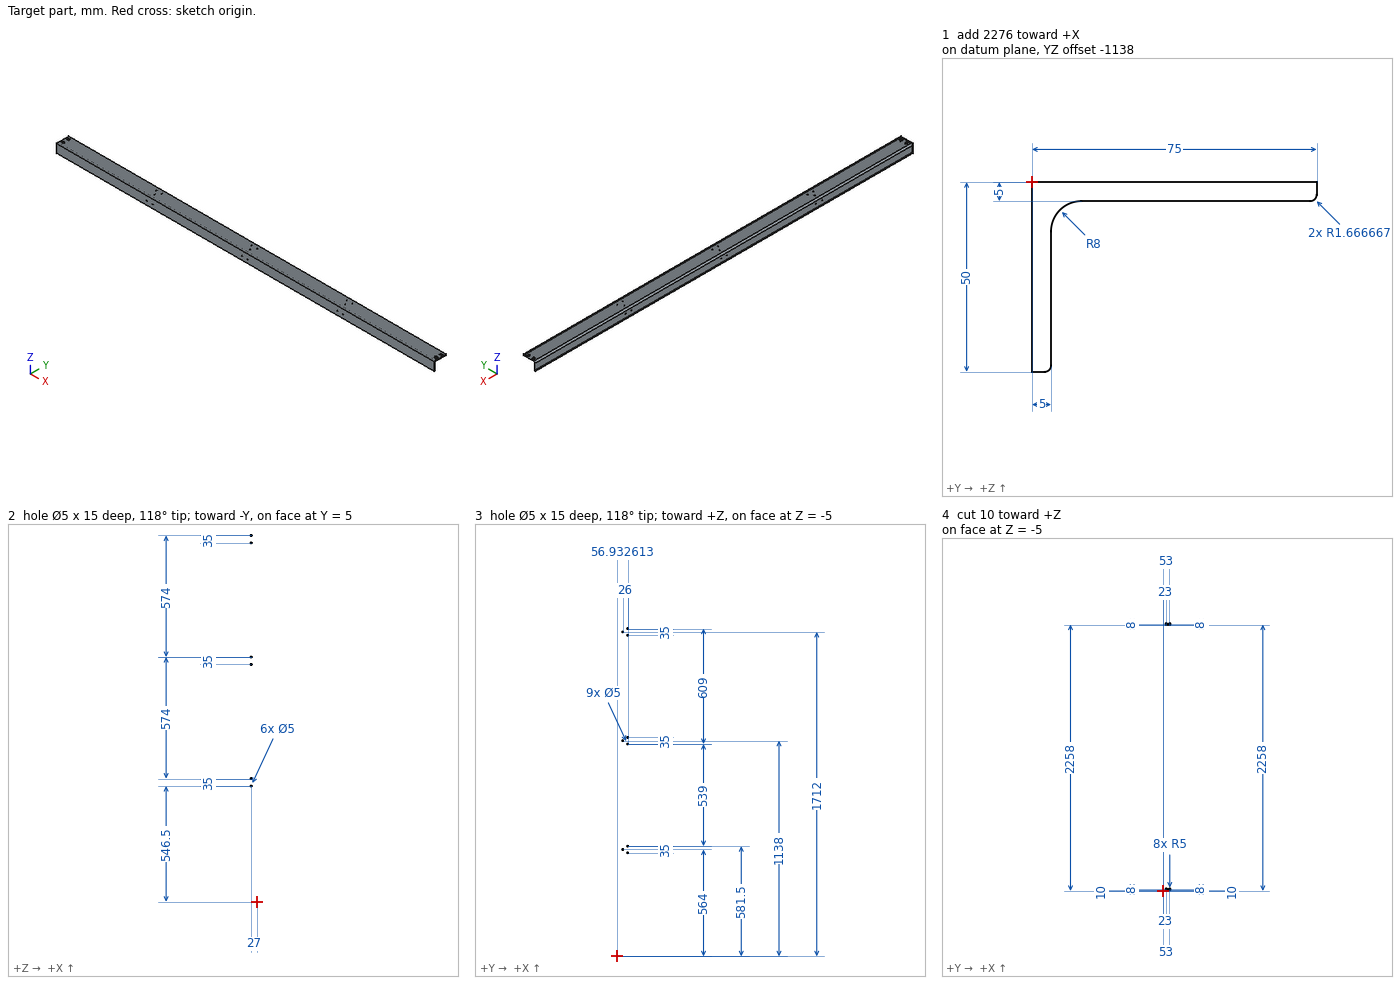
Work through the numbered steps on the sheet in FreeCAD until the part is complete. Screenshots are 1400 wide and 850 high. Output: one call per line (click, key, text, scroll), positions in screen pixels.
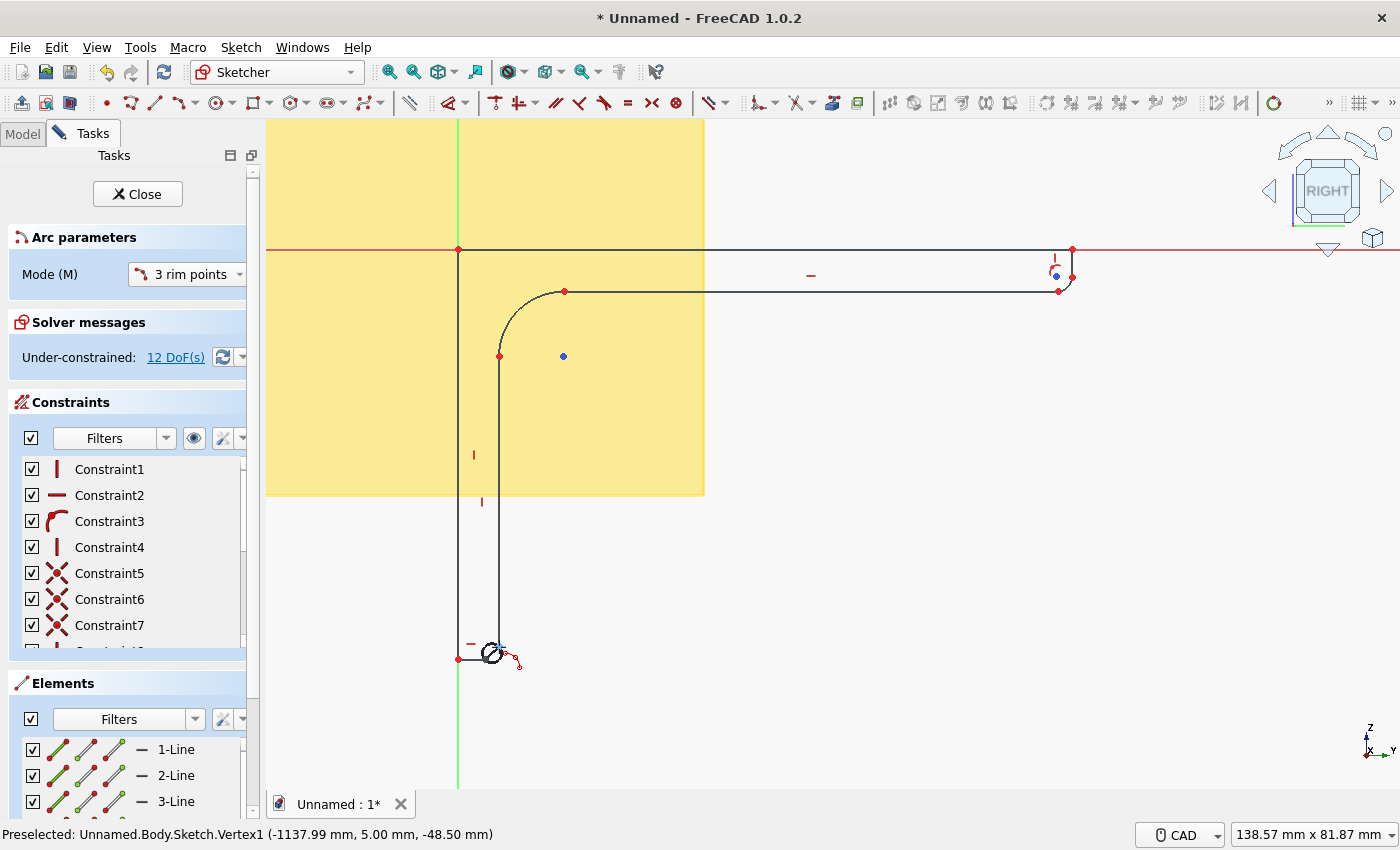
scroll(495, 655, up, 7)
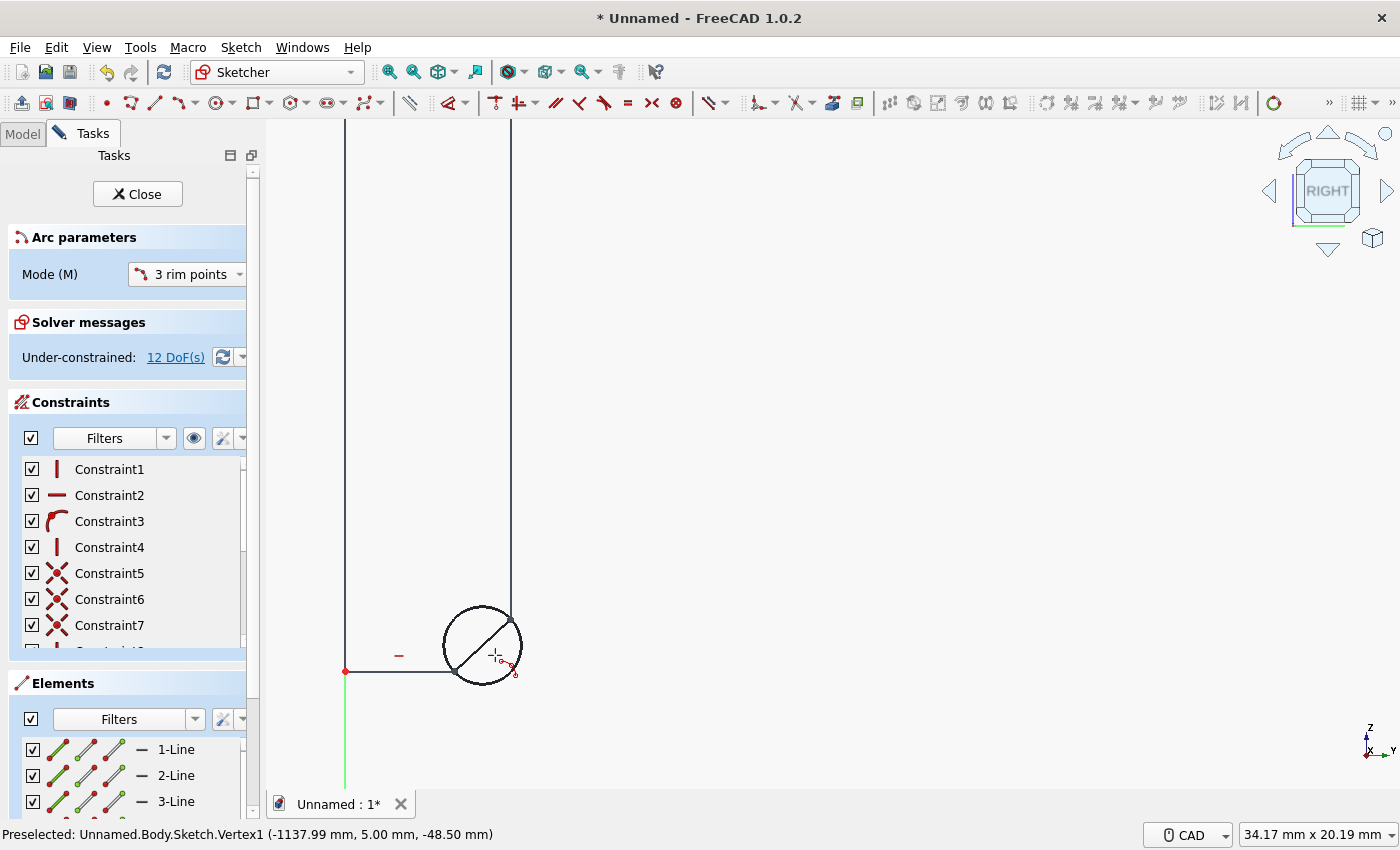
click(495, 653)
key(Escape)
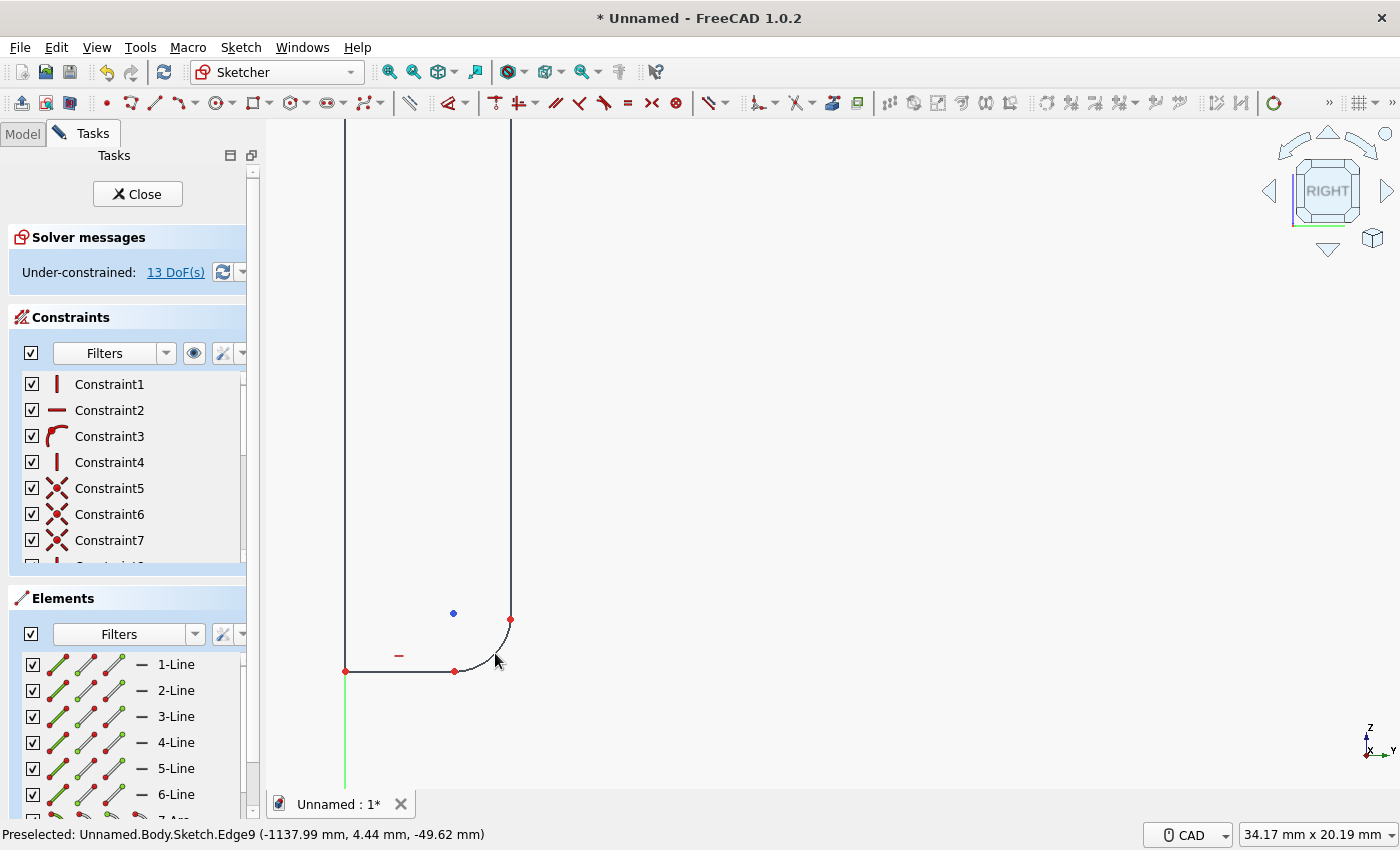
scroll(494, 655, down, 7)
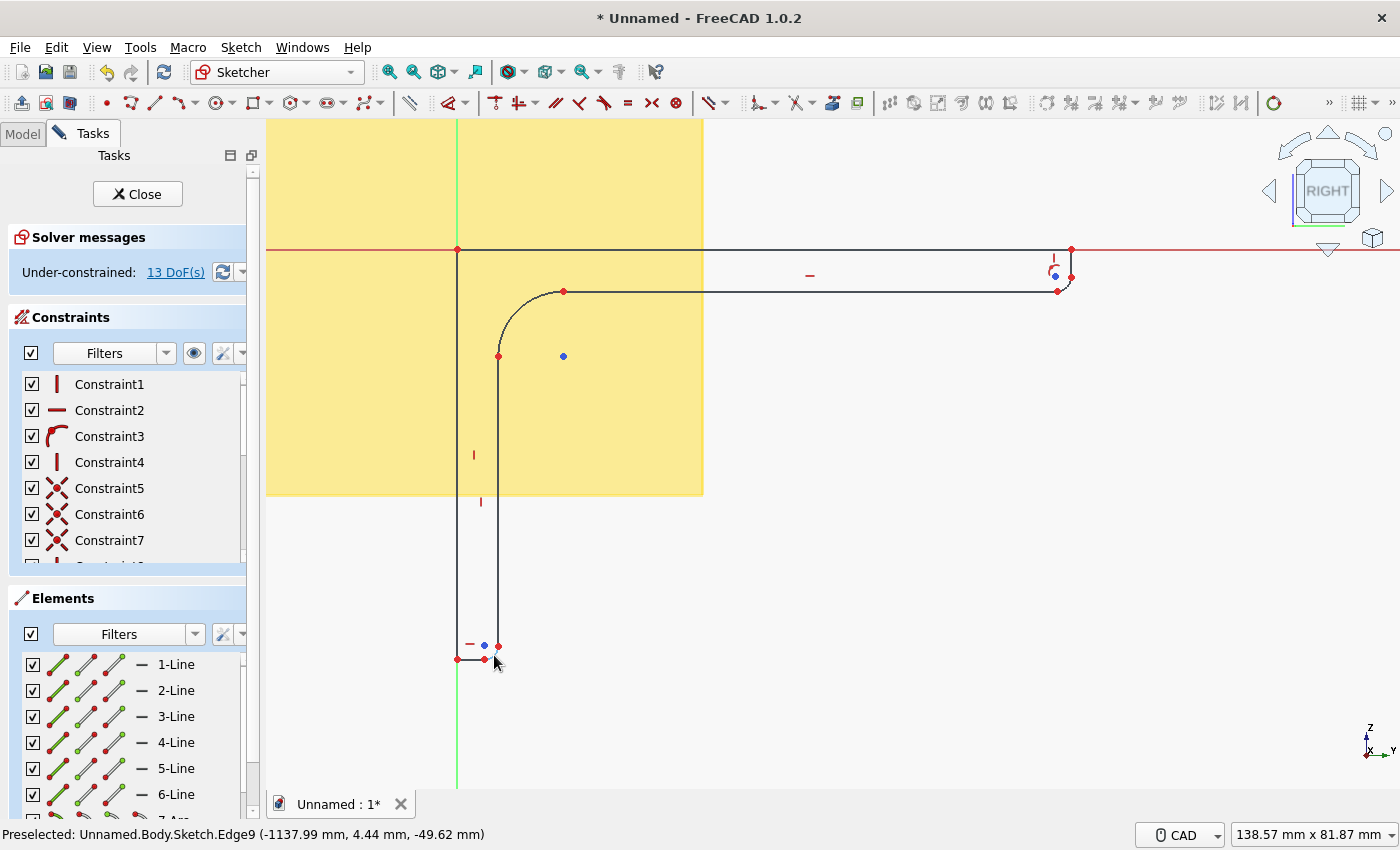
click(498, 560)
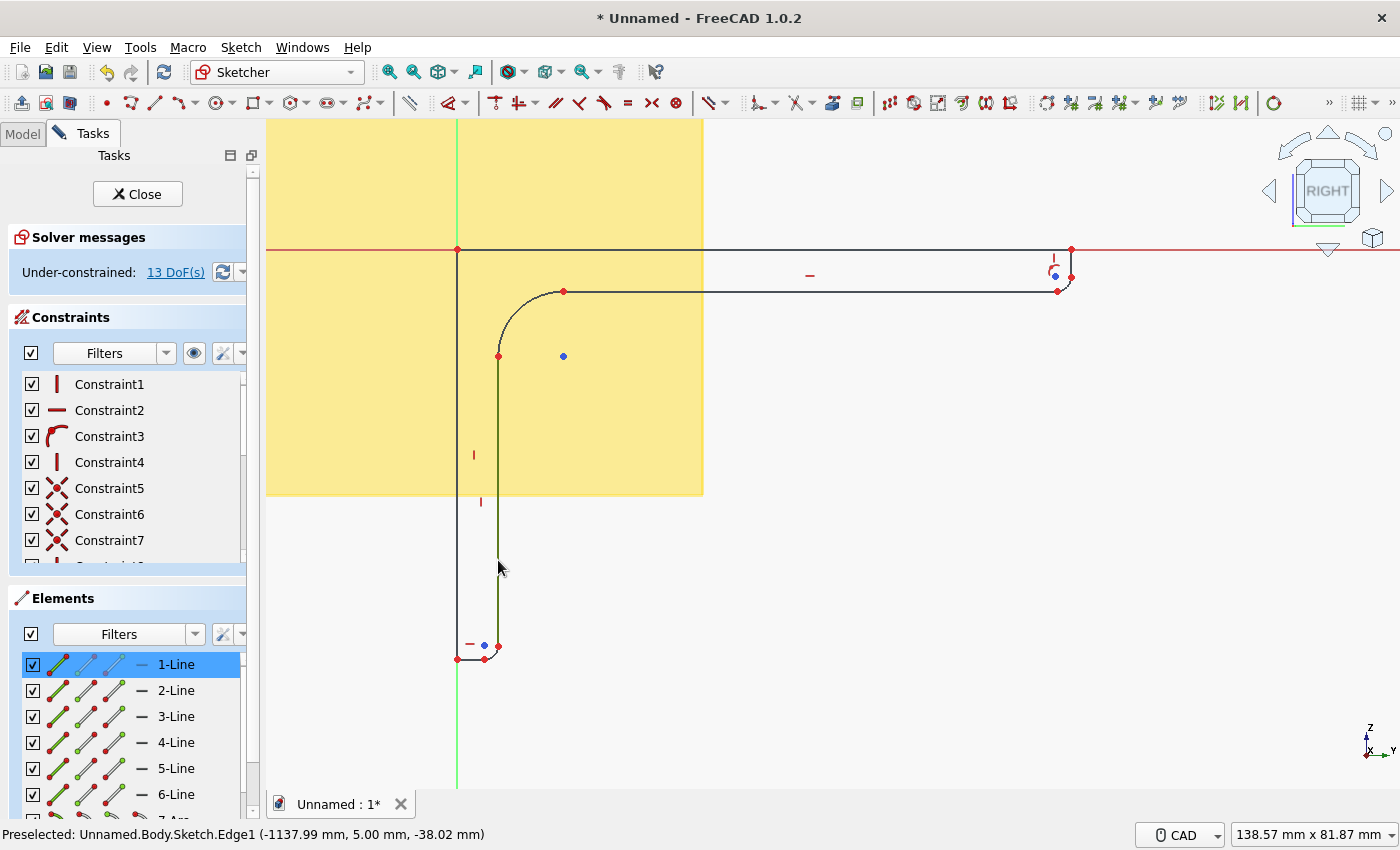
click(534, 299)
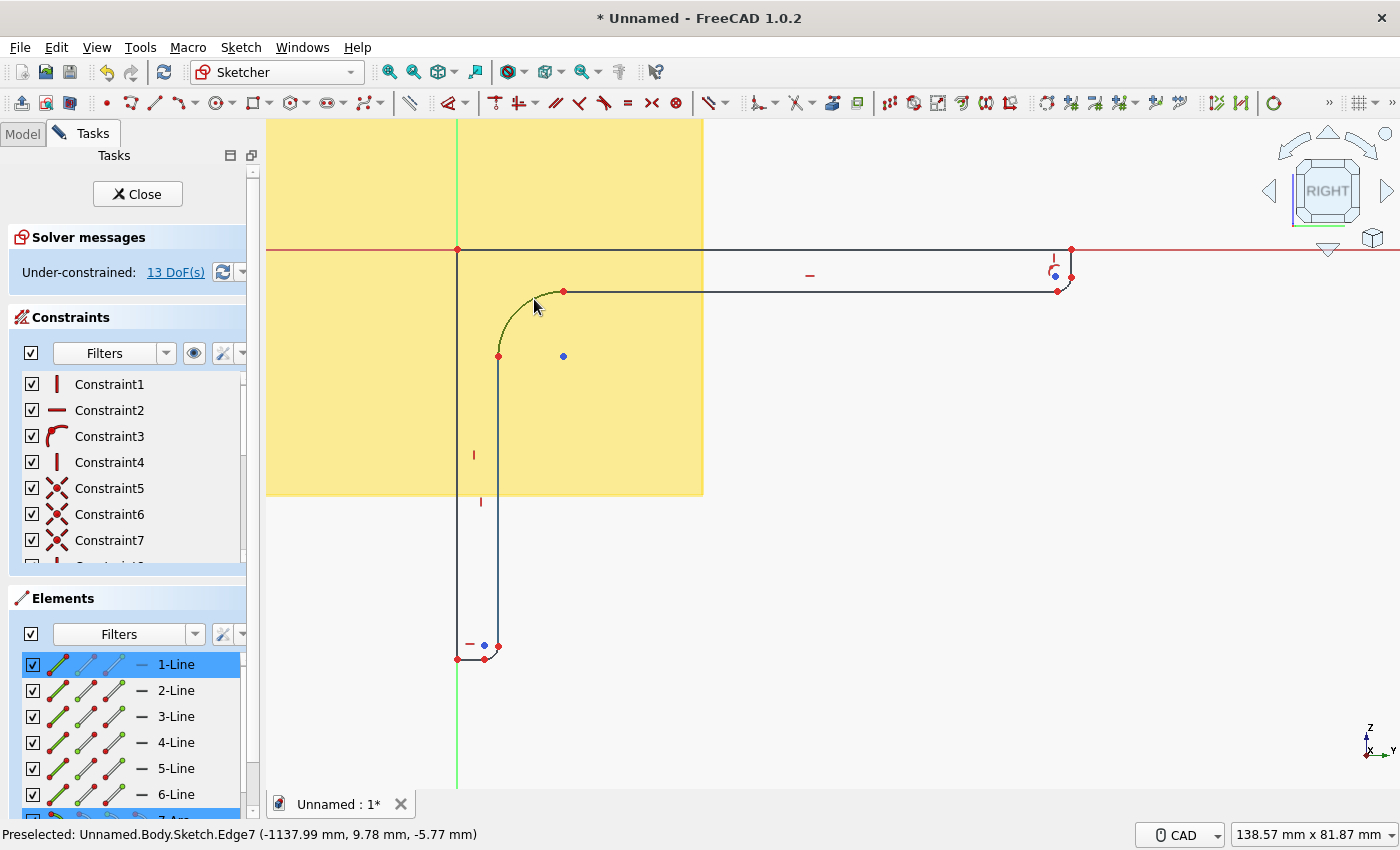
click(604, 104)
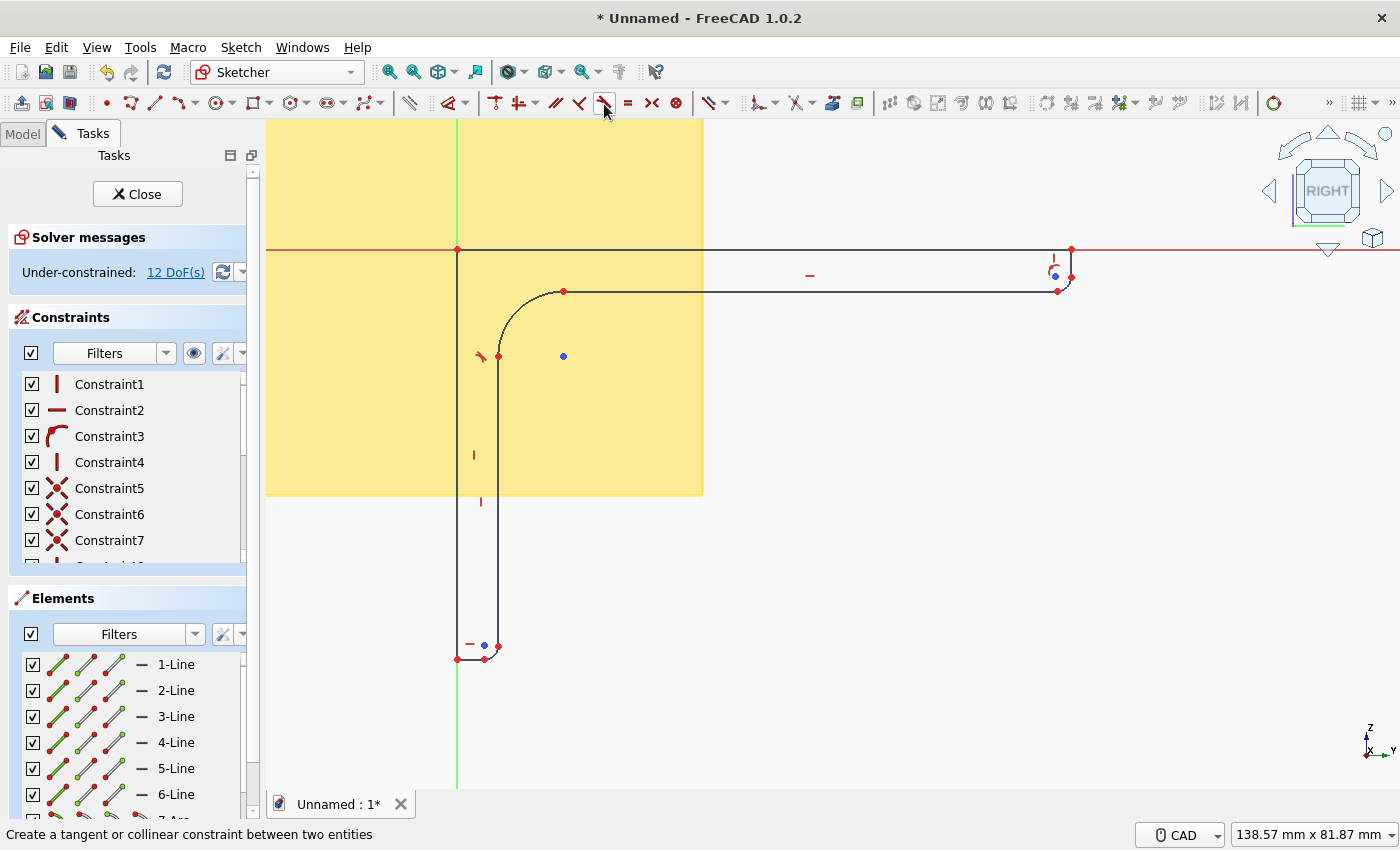
click(498, 560)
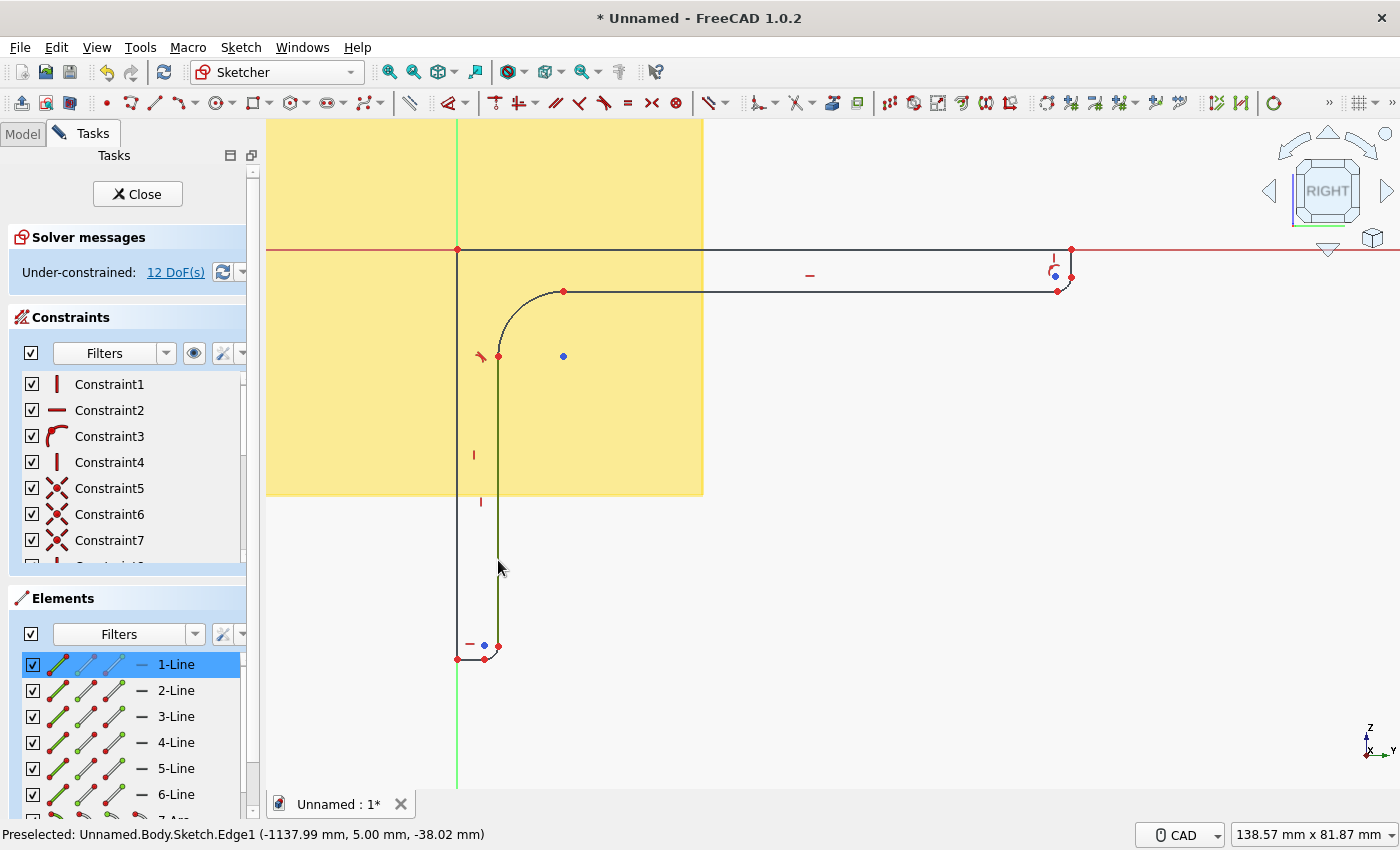
scroll(494, 656, up, 2)